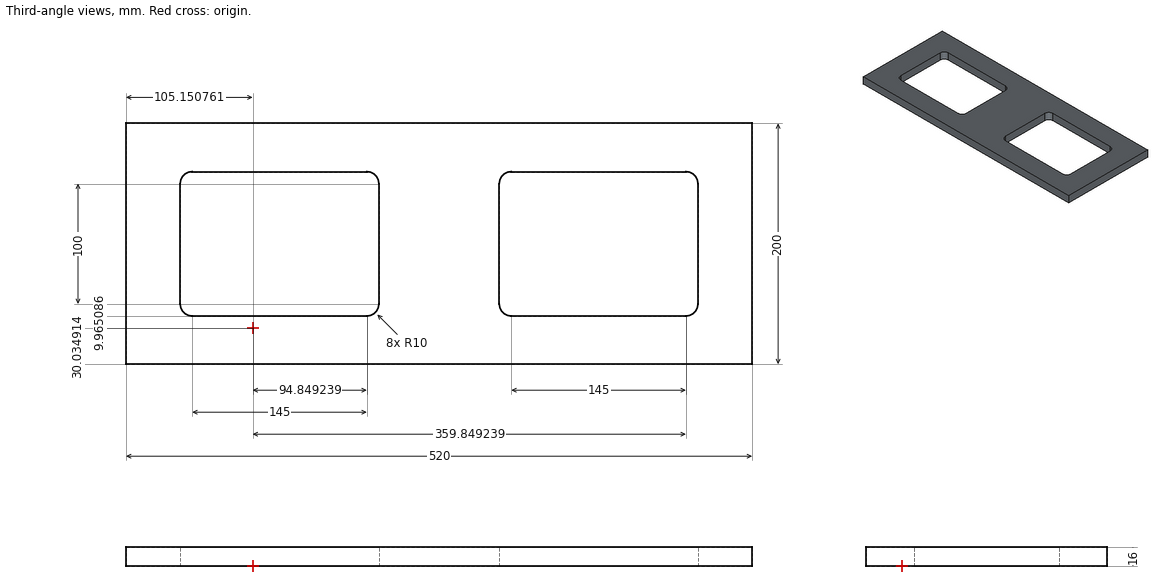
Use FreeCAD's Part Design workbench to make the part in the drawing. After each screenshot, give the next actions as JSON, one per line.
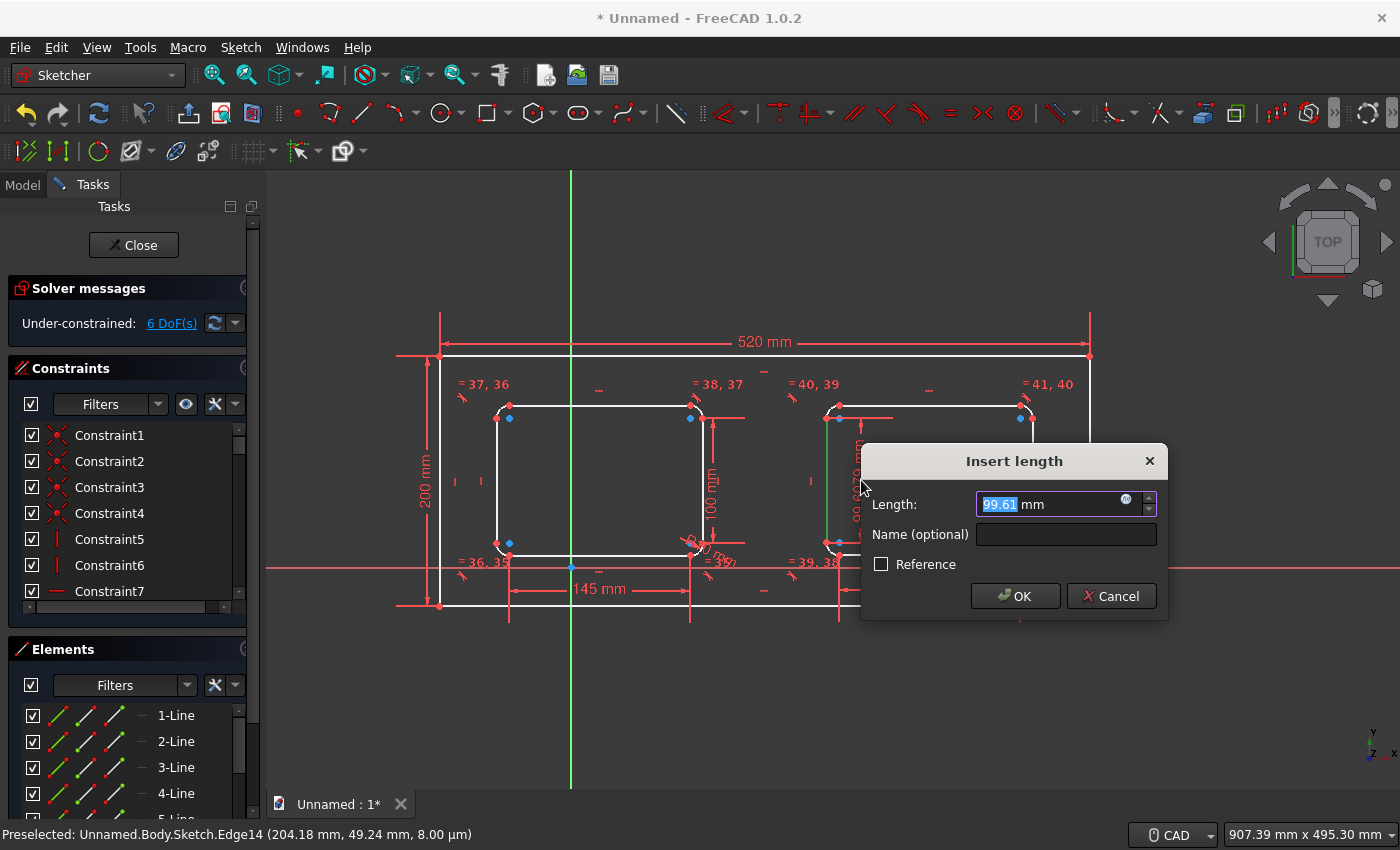
{"action": "type", "text": "100"}
{"action": "key", "text": "Return"}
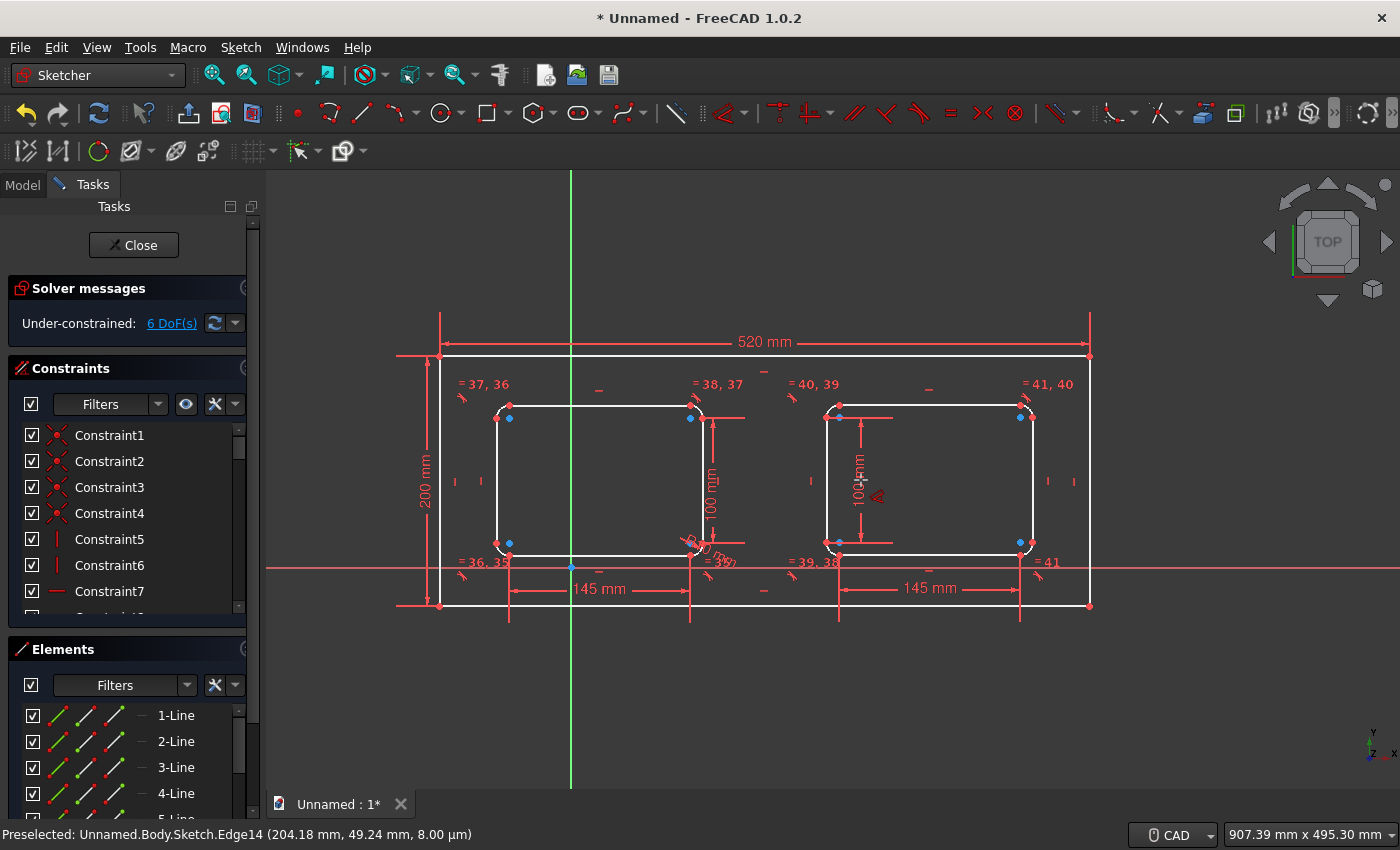
{"action": "scroll", "coordinate": [690, 556], "scroll_direction": "up", "scroll_amount": 6}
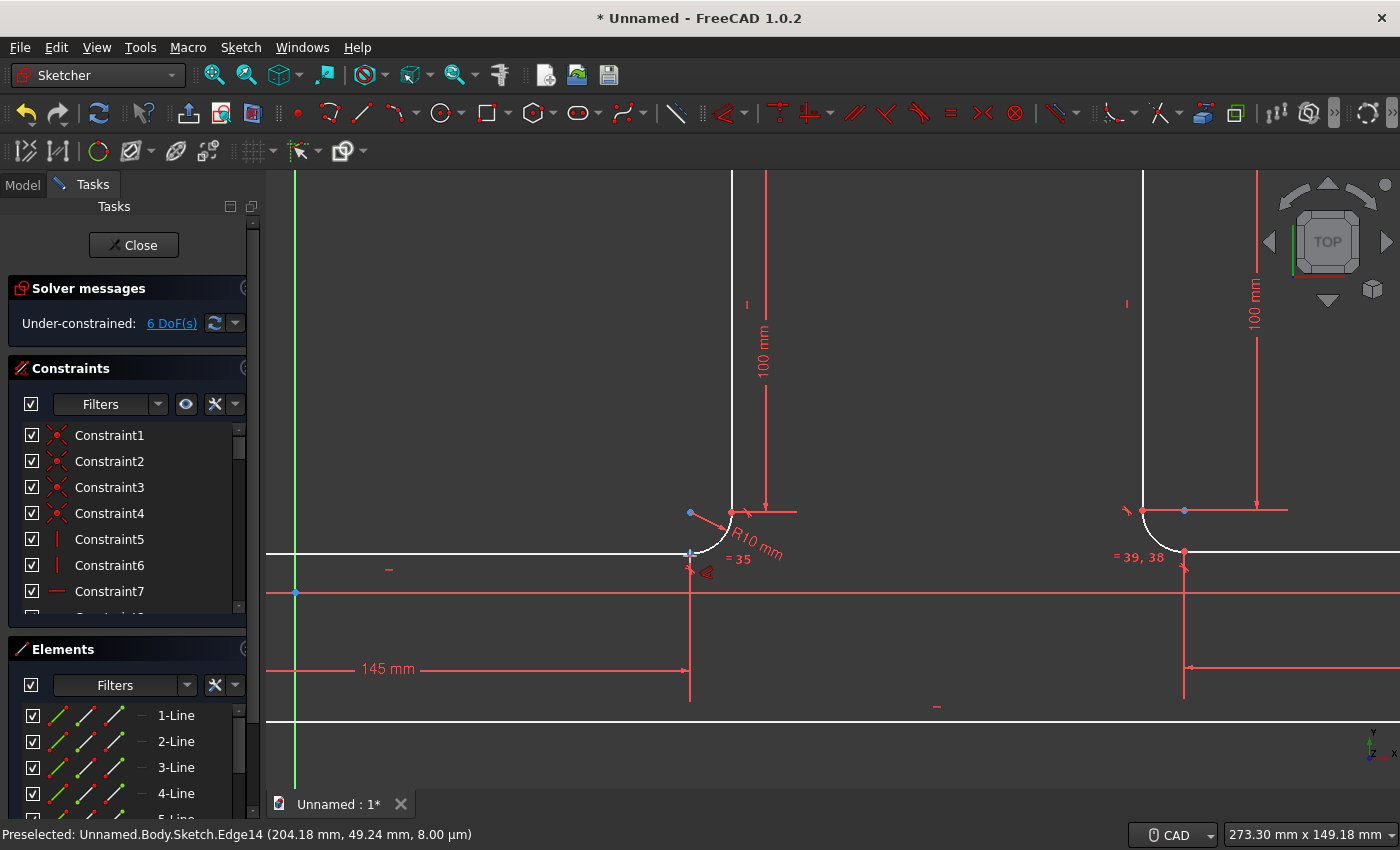
{"action": "left_click", "coordinate": [690, 554]}
{"action": "left_click", "coordinate": [724, 573]}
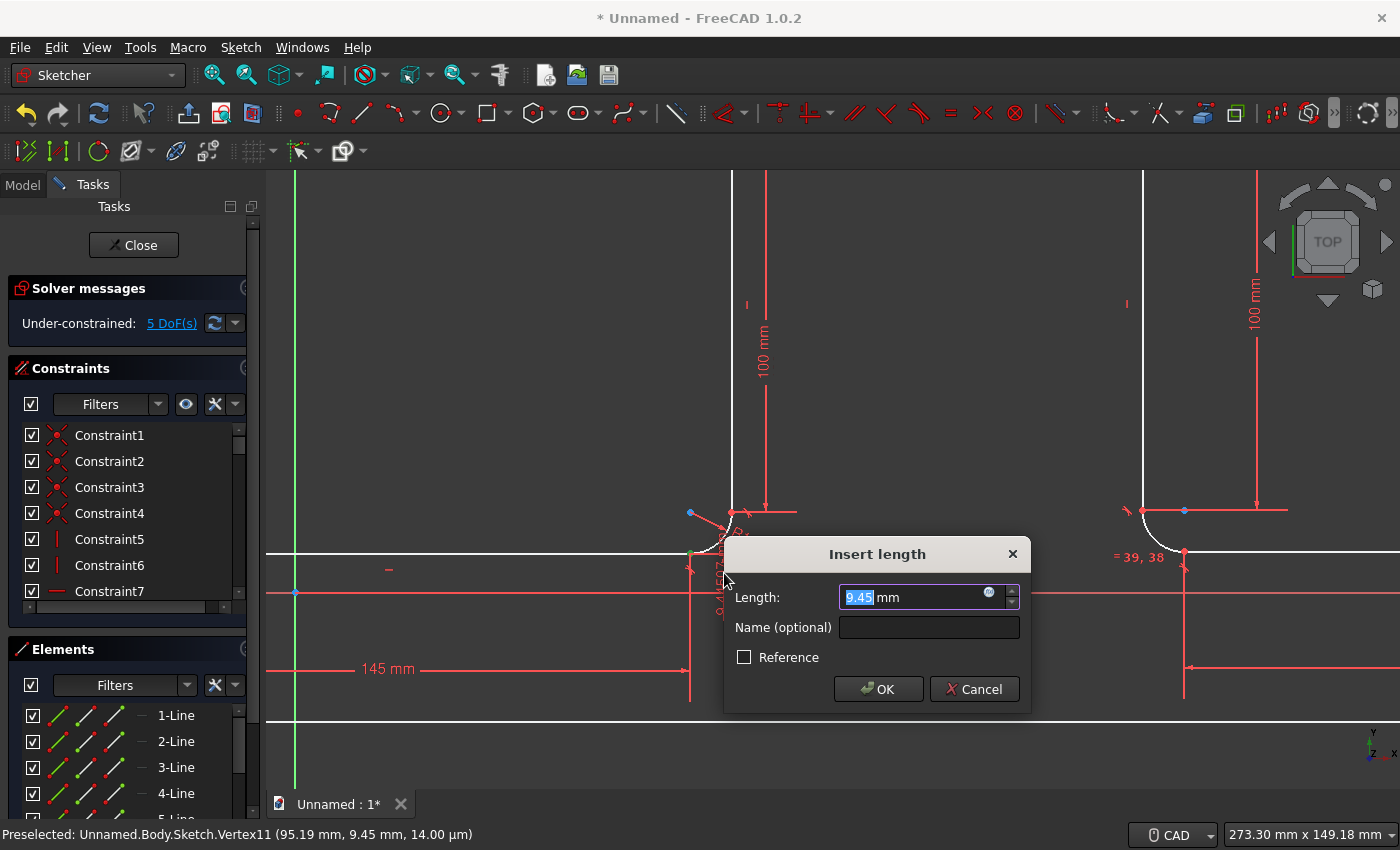
{"action": "type", "text": "9.965086"}
{"action": "key", "text": "Return"}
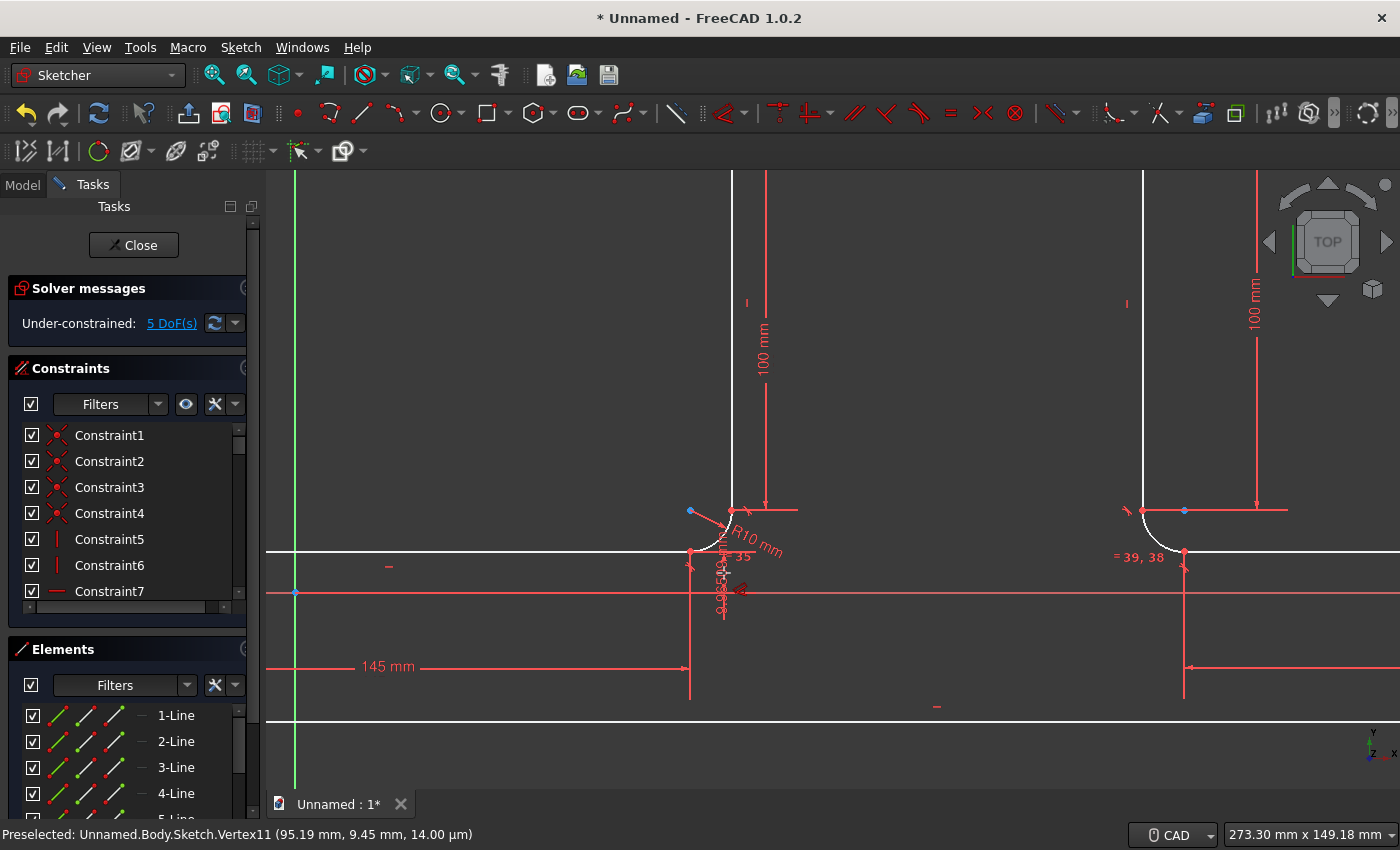
{"action": "scroll", "coordinate": [690, 556], "scroll_direction": "down", "scroll_amount": 6}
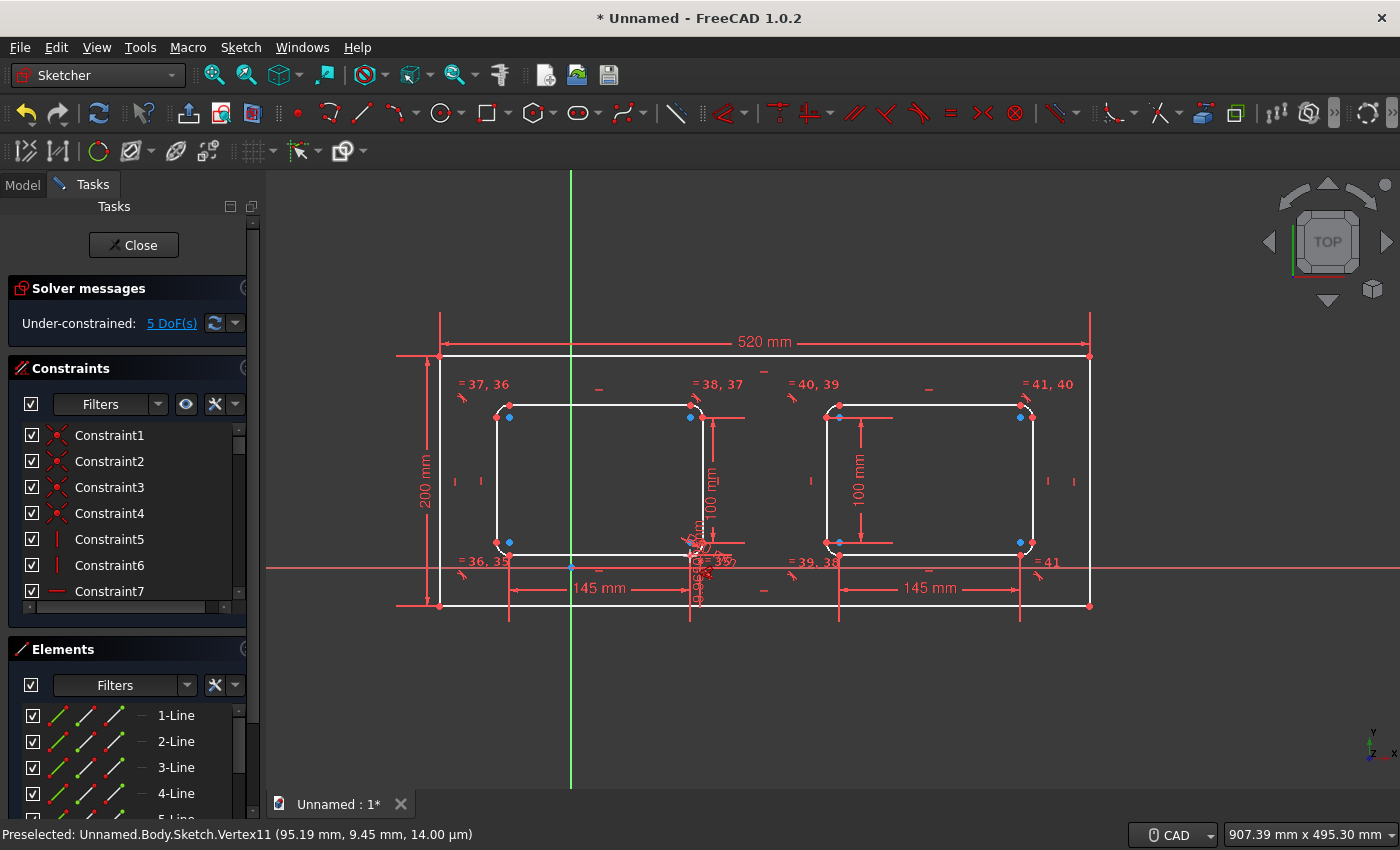
{"action": "scroll", "coordinate": [1020, 555], "scroll_direction": "up", "scroll_amount": 6}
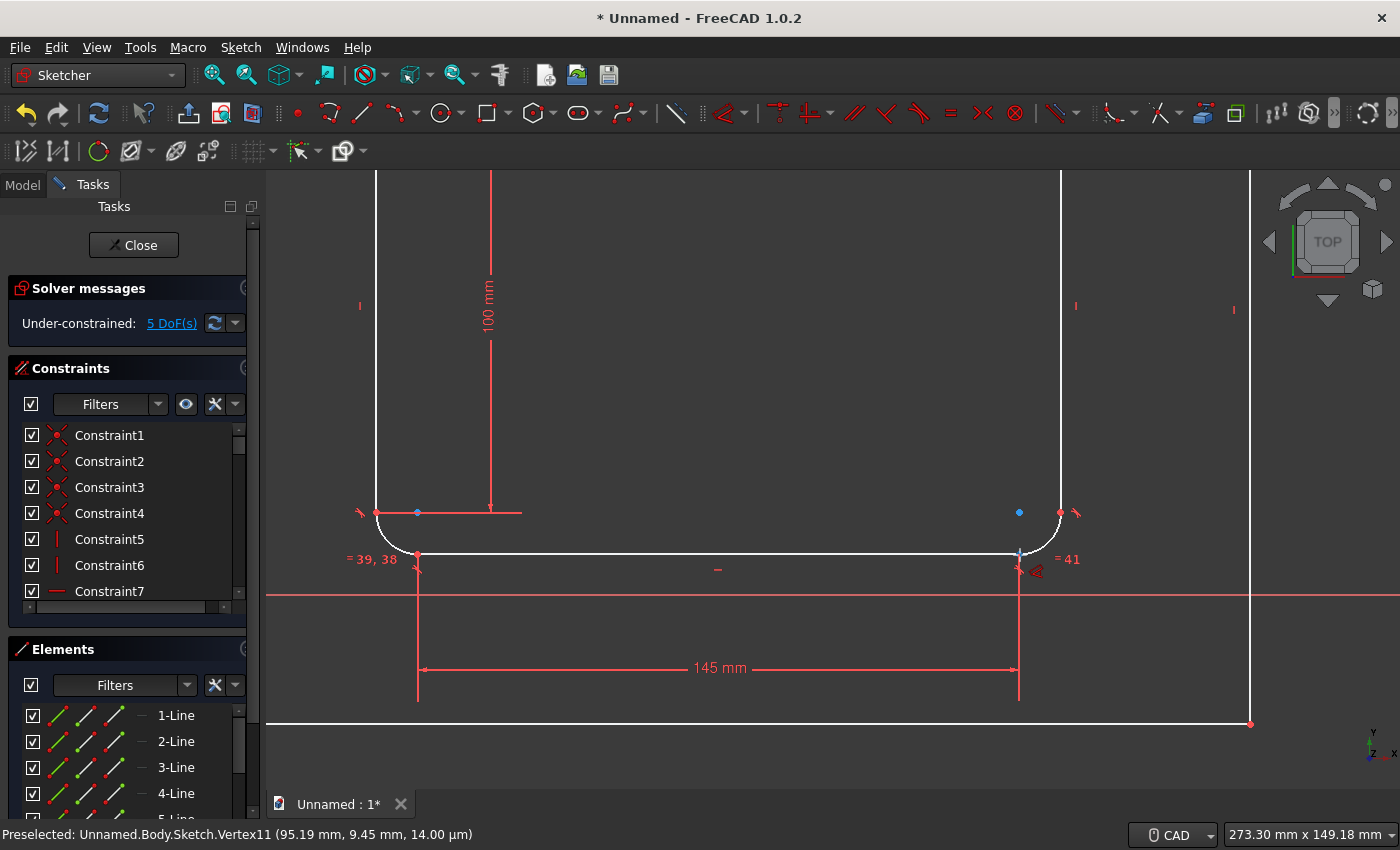
{"action": "left_click", "coordinate": [1019, 554]}
{"action": "left_click", "coordinate": [1053, 575]}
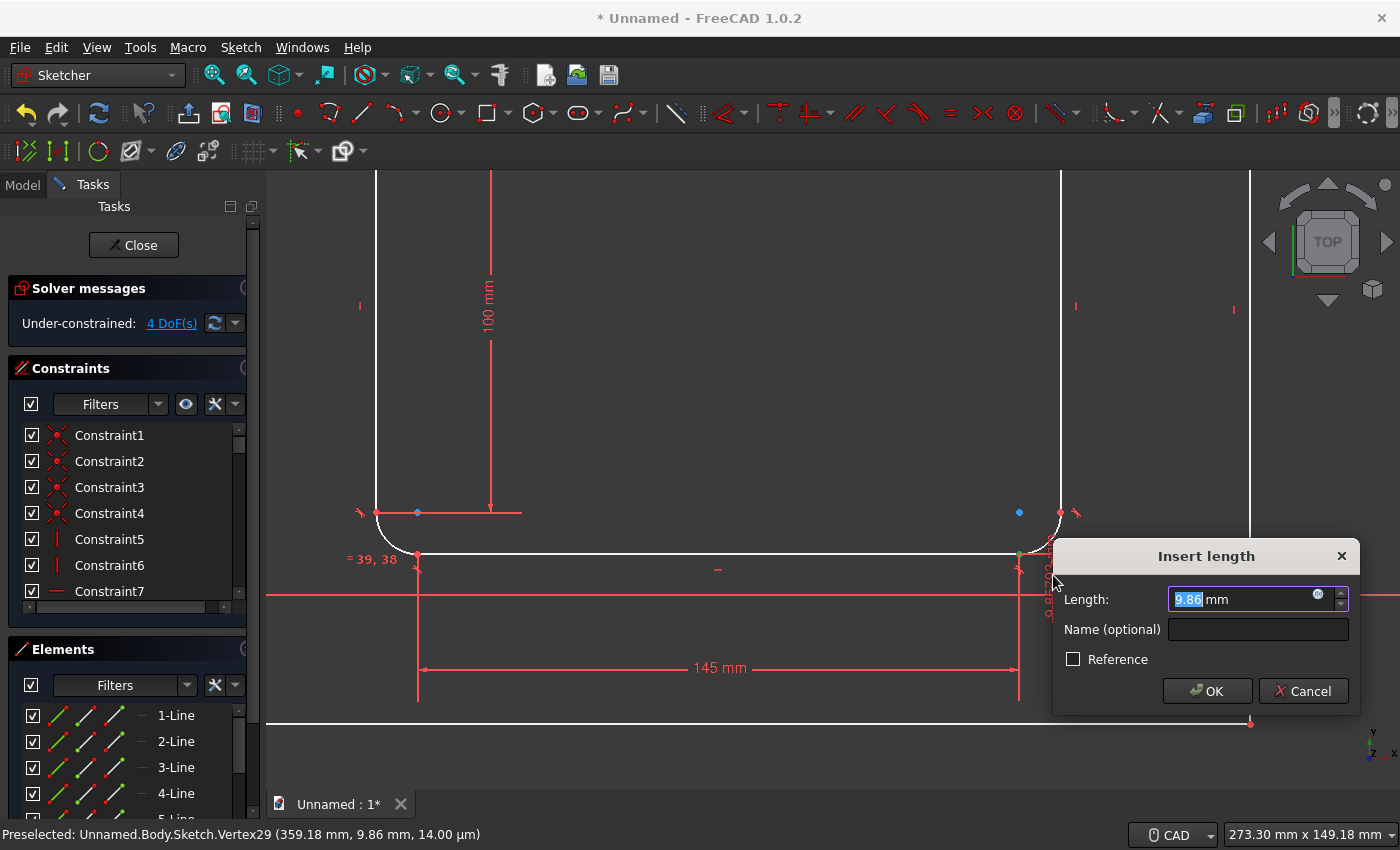
{"action": "type", "text": "9.965086"}
{"action": "key", "text": "Return"}